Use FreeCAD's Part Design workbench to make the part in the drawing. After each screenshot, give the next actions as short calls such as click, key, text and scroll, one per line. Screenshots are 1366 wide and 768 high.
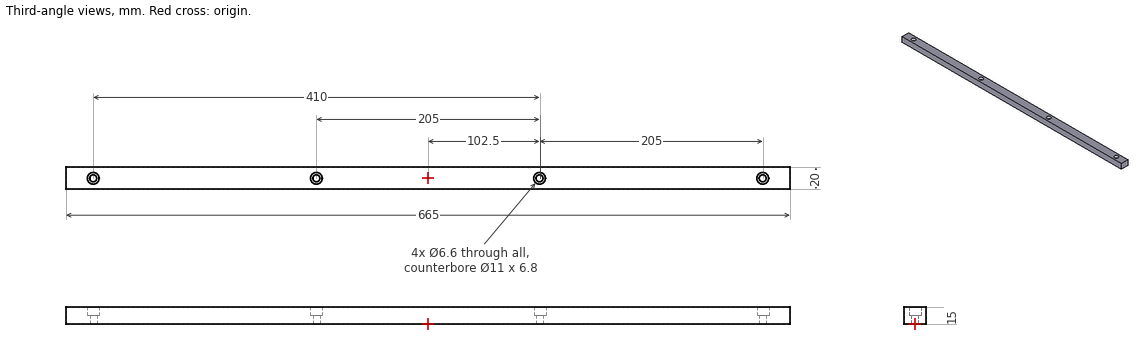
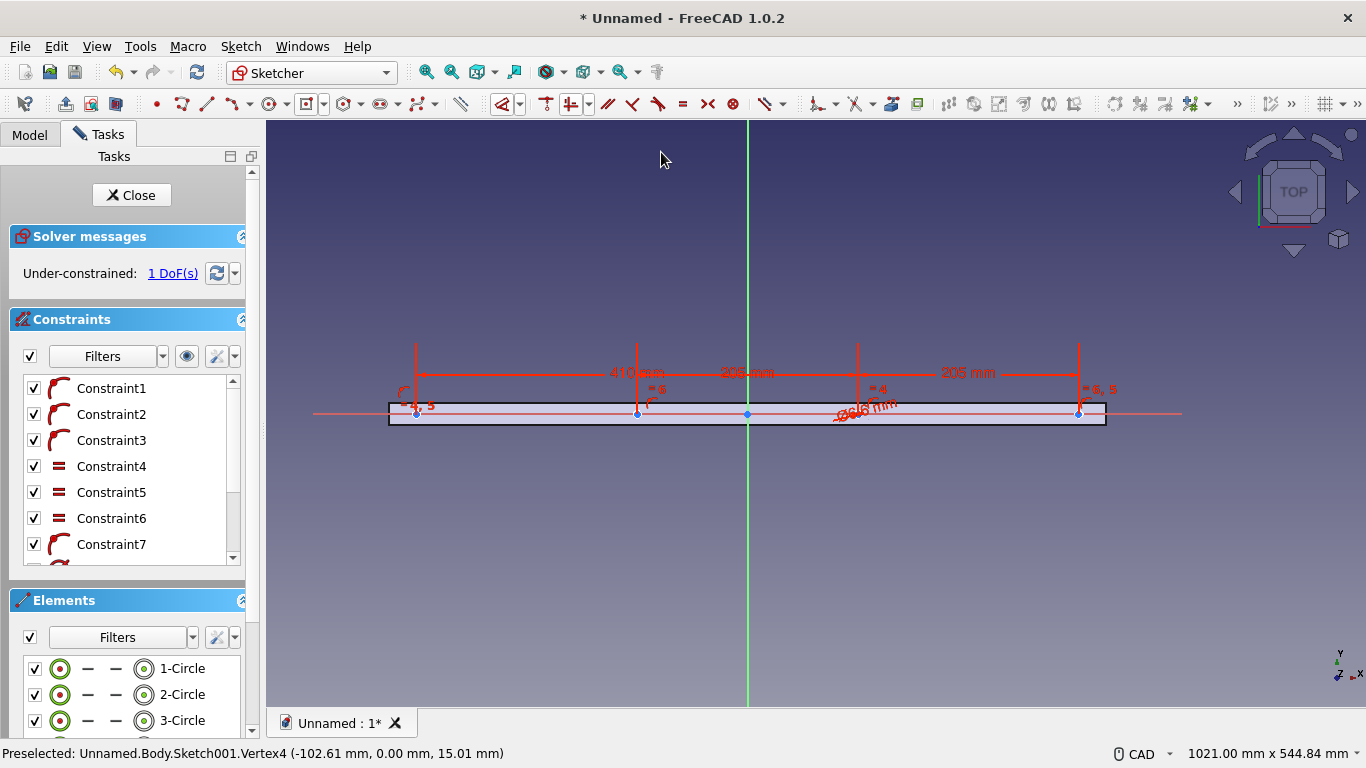
click(858, 414)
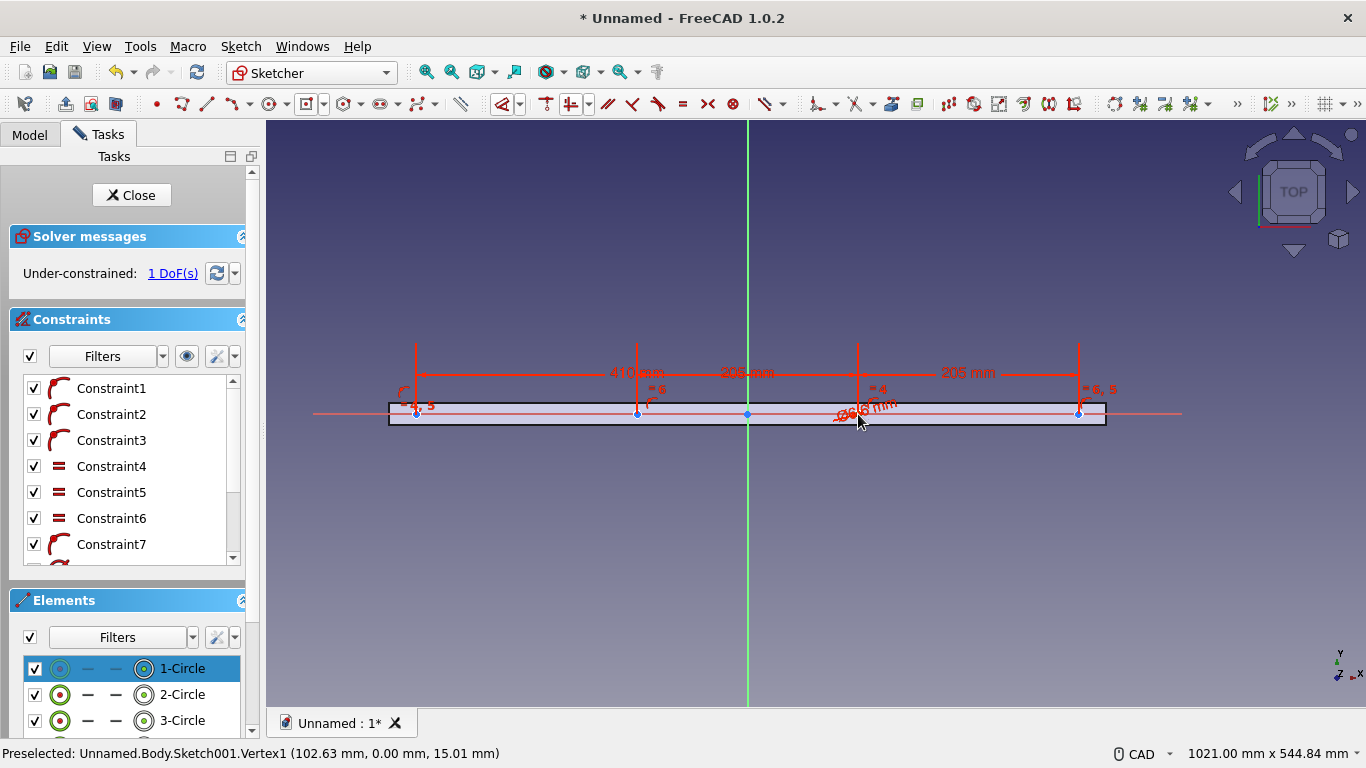
click(520, 104)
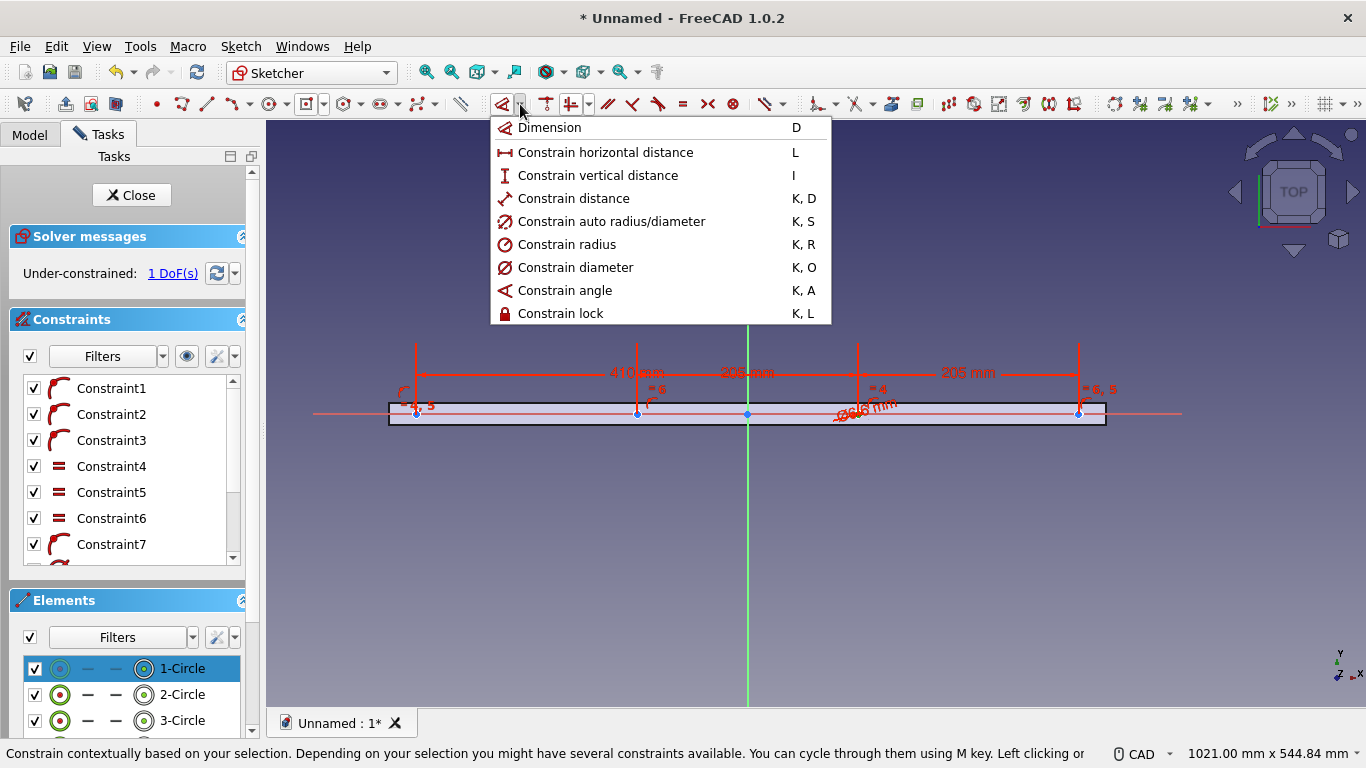
click(661, 152)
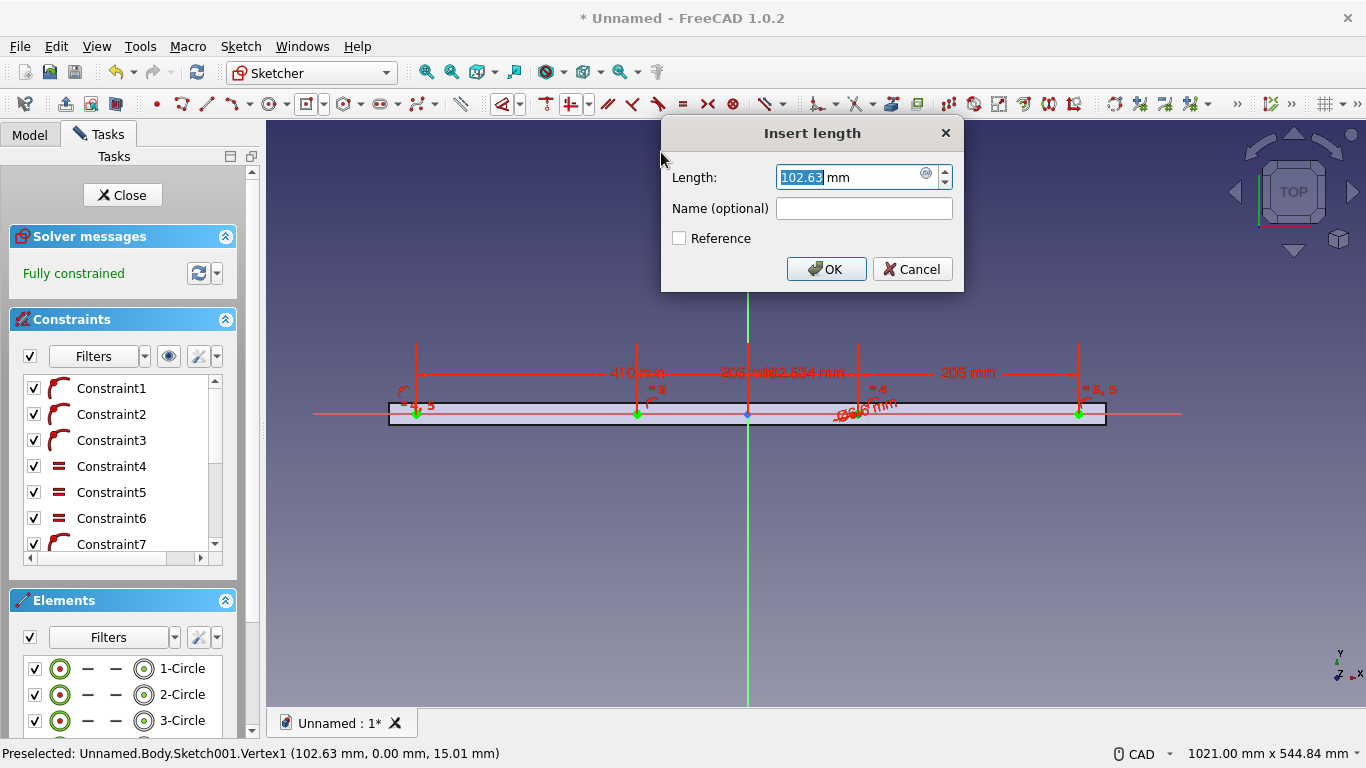
text(102.5)
key(Return)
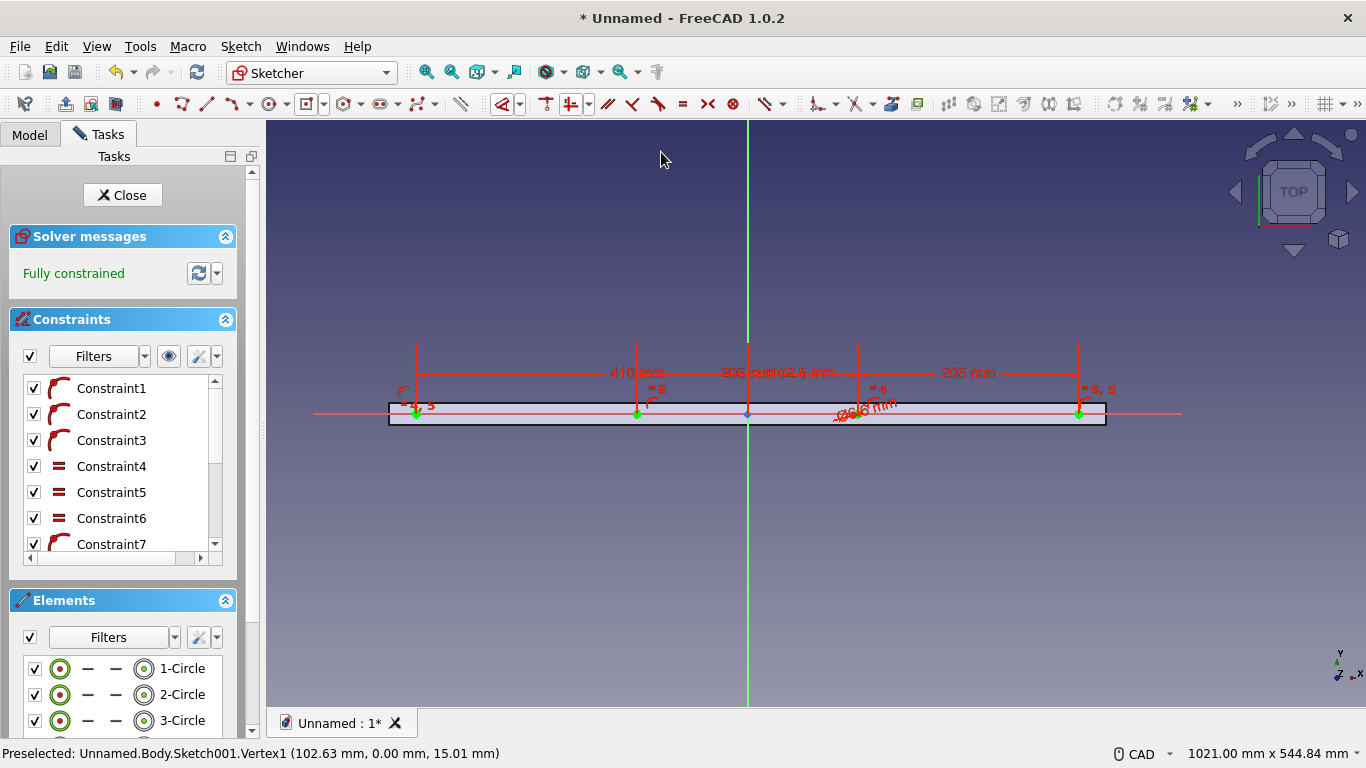
click(123, 195)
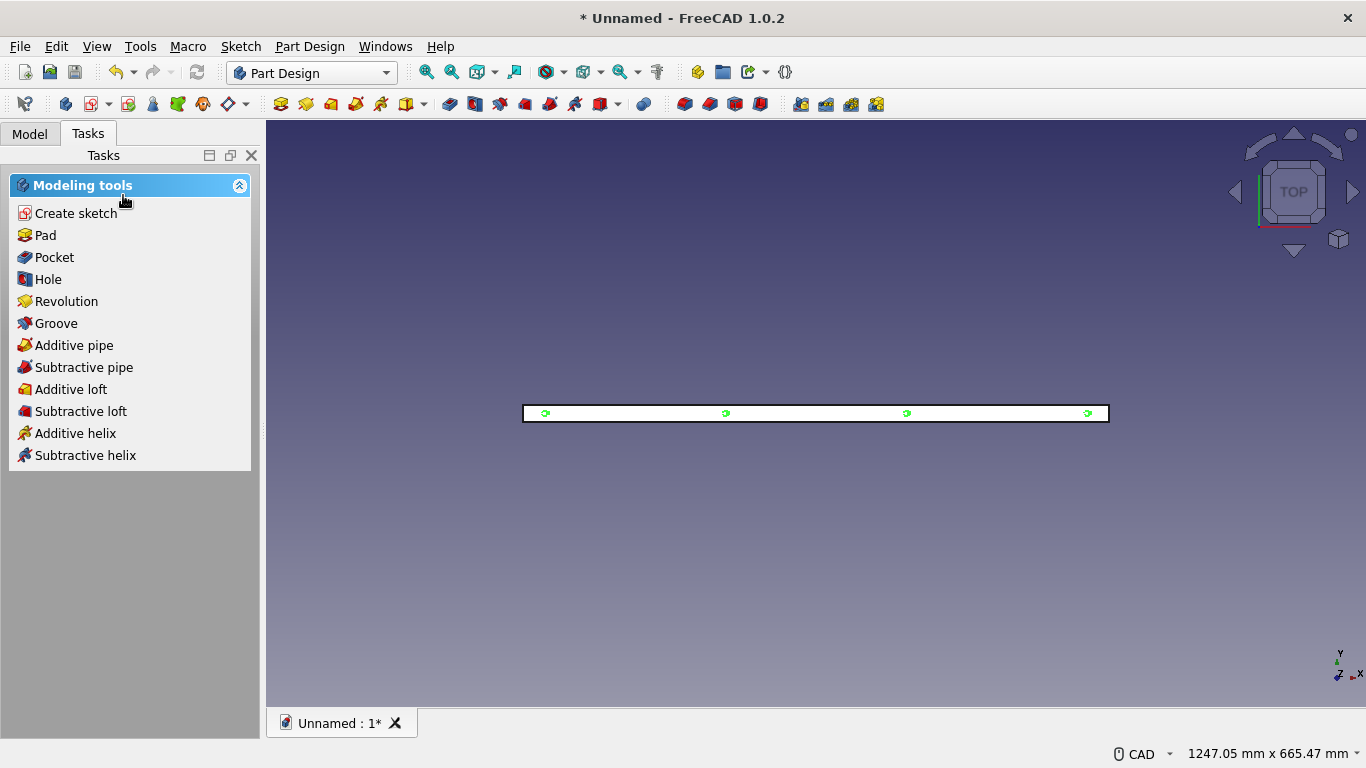
click(475, 104)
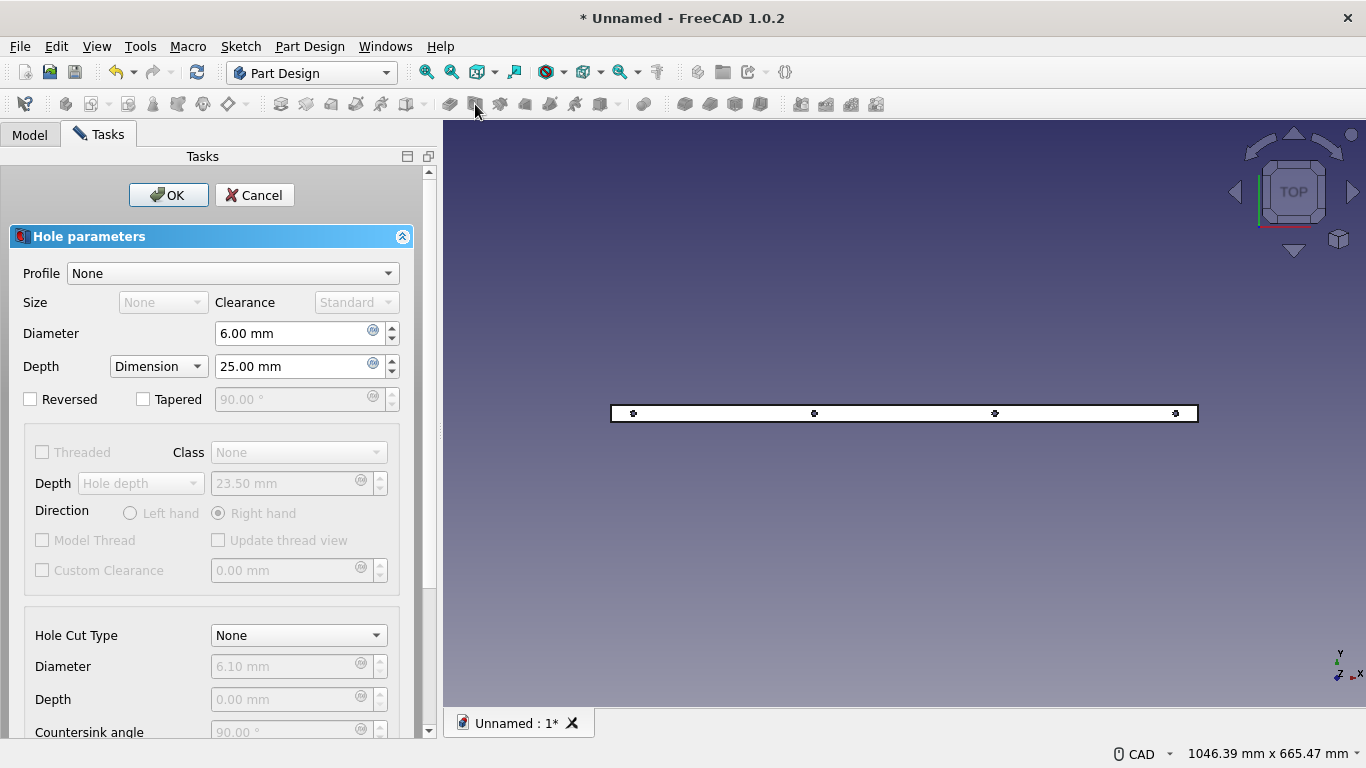
triple_click(300, 334)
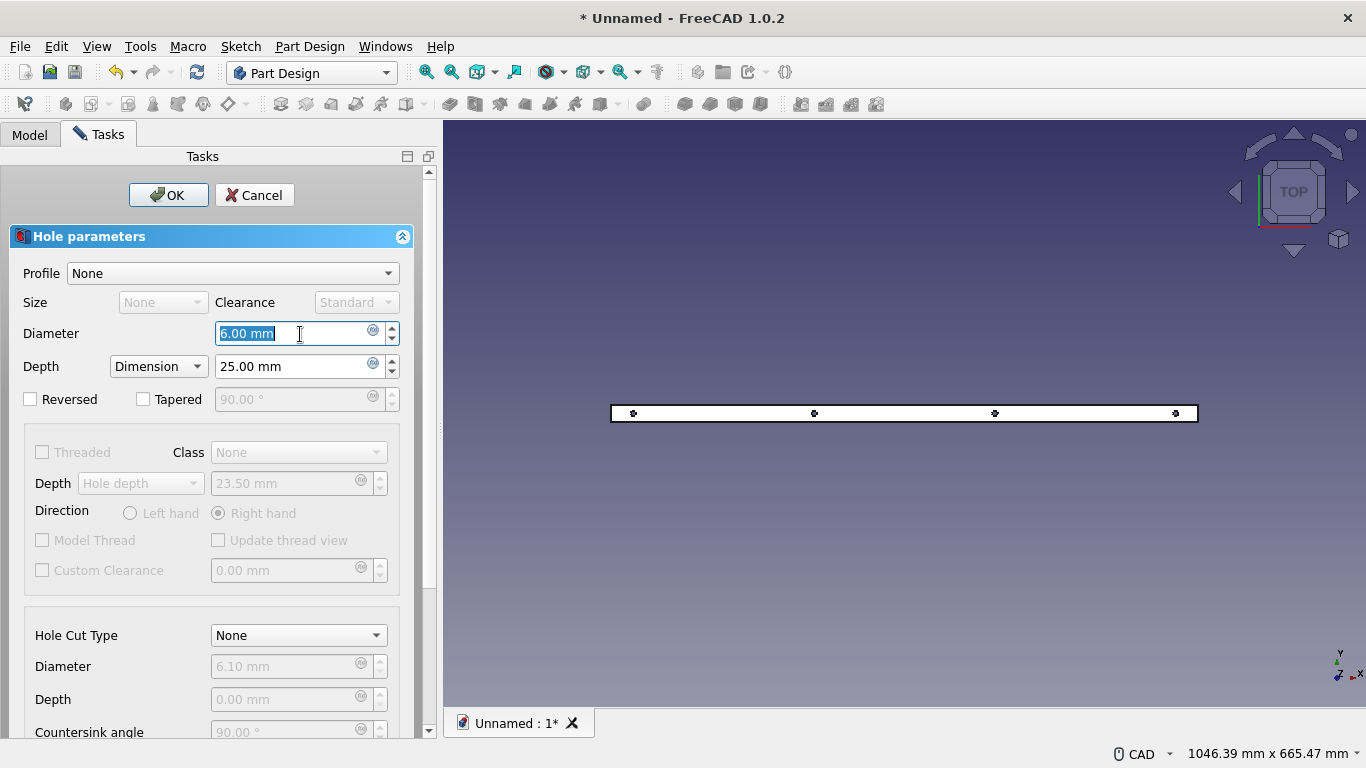
text(6.6)
key(Tab)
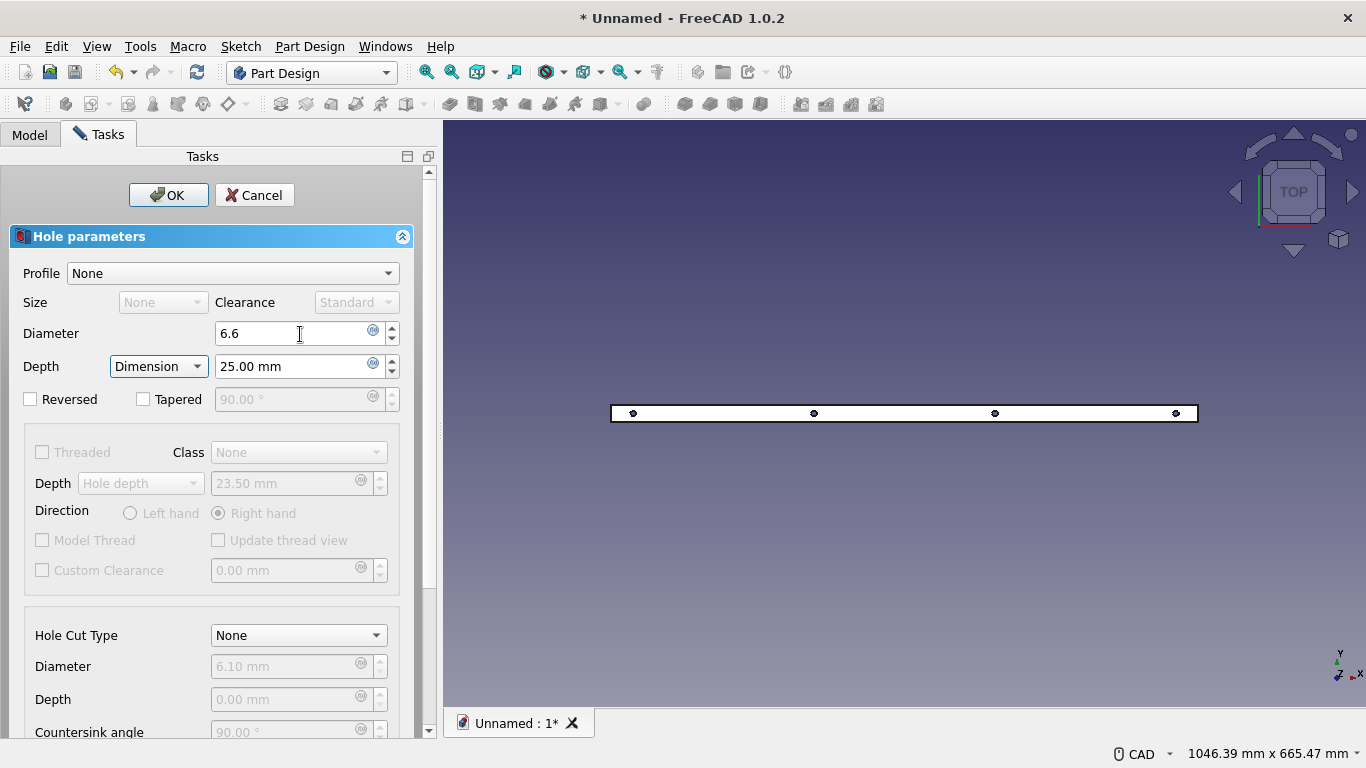
click(160, 366)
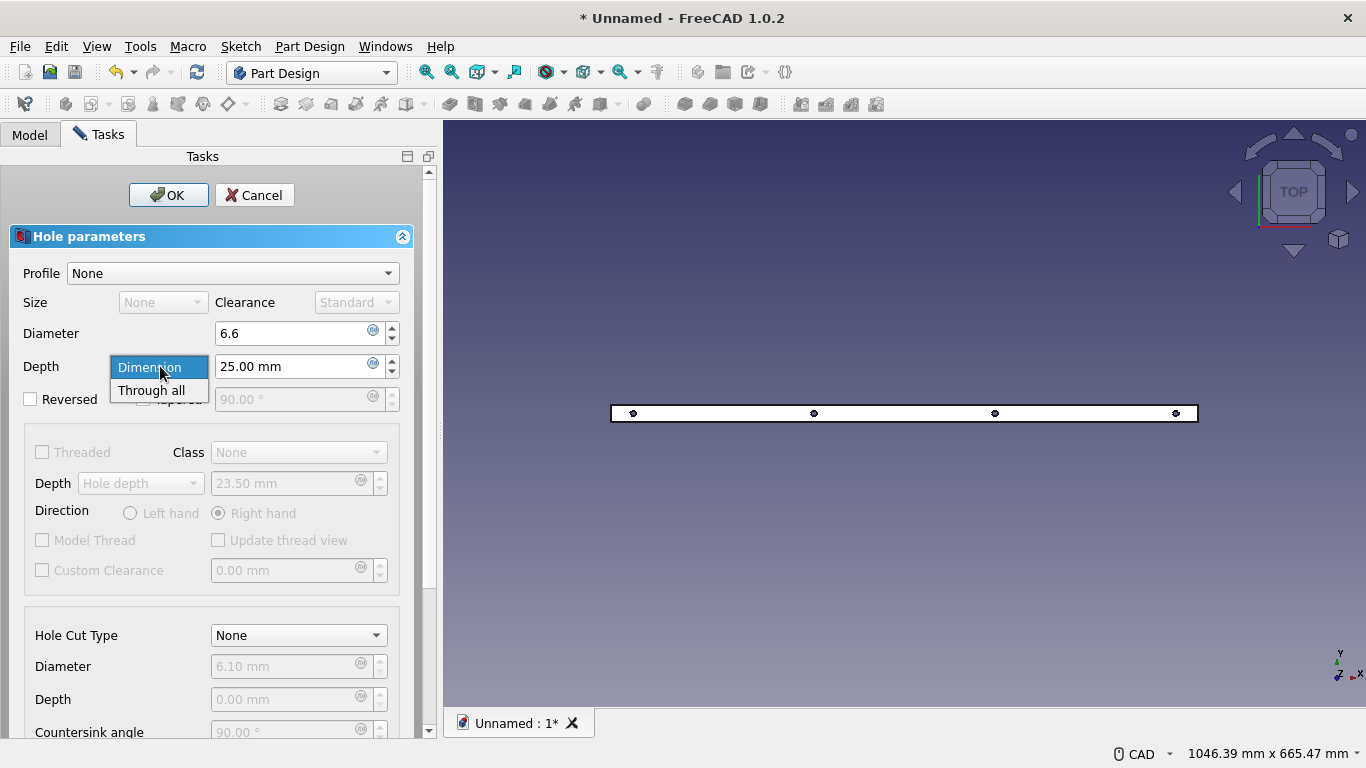
click(158, 390)